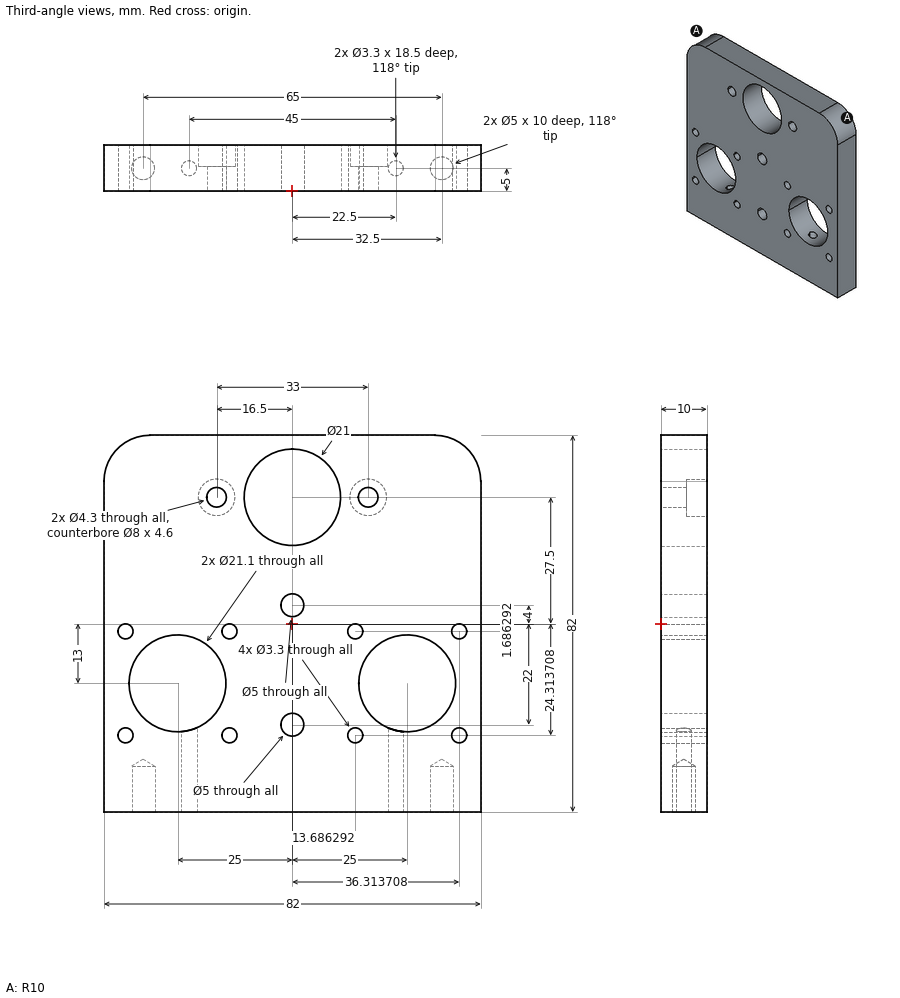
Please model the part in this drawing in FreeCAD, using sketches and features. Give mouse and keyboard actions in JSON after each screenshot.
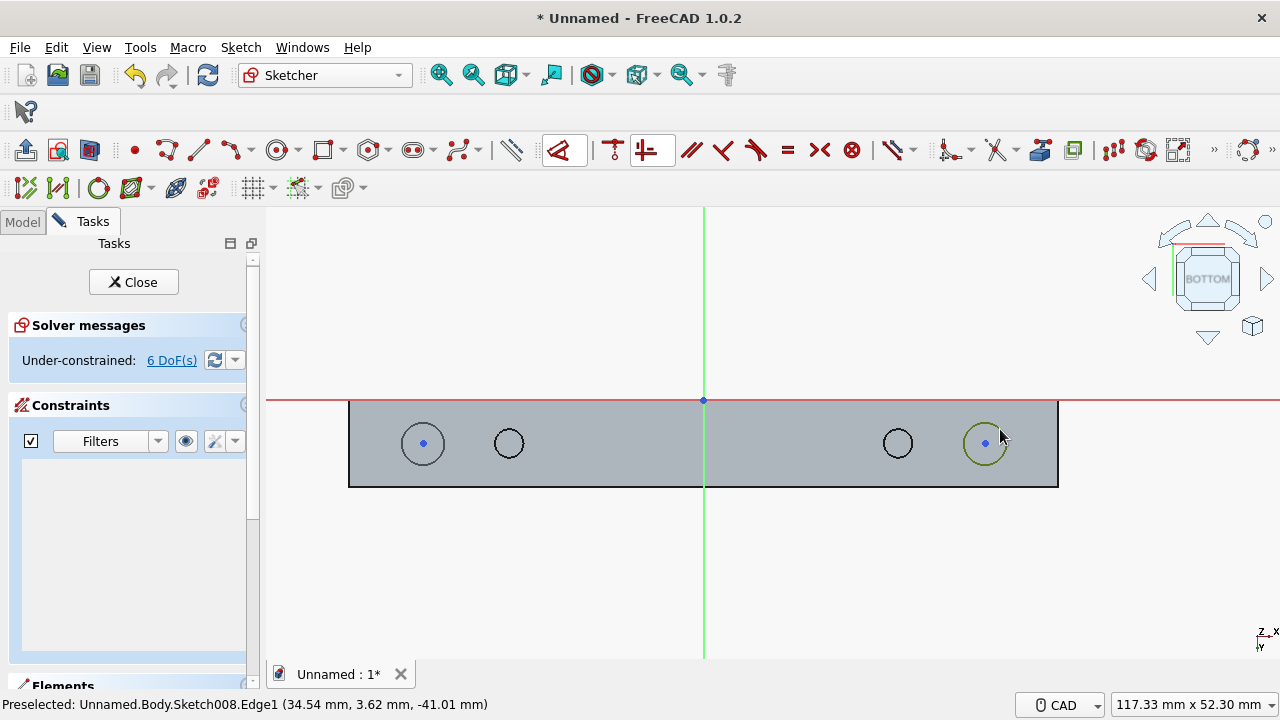
{"action": "left_click", "coordinate": [438, 429]}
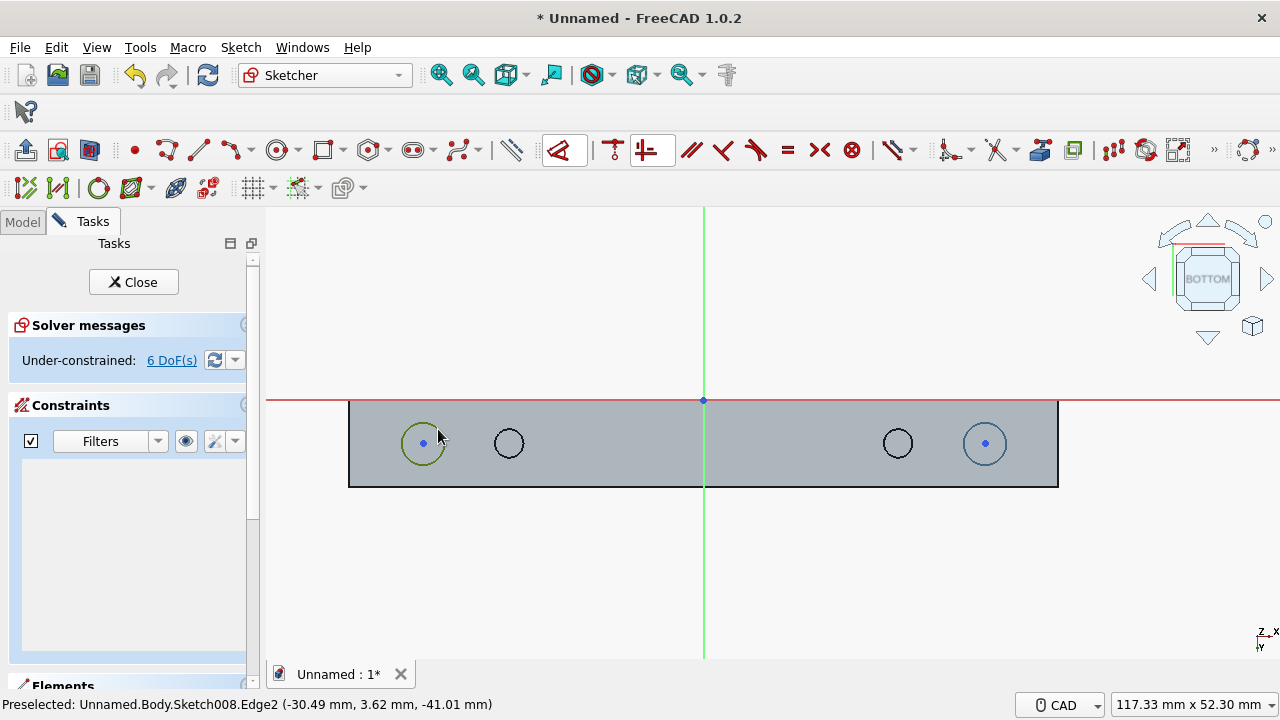
{"action": "left_click", "coordinate": [788, 150]}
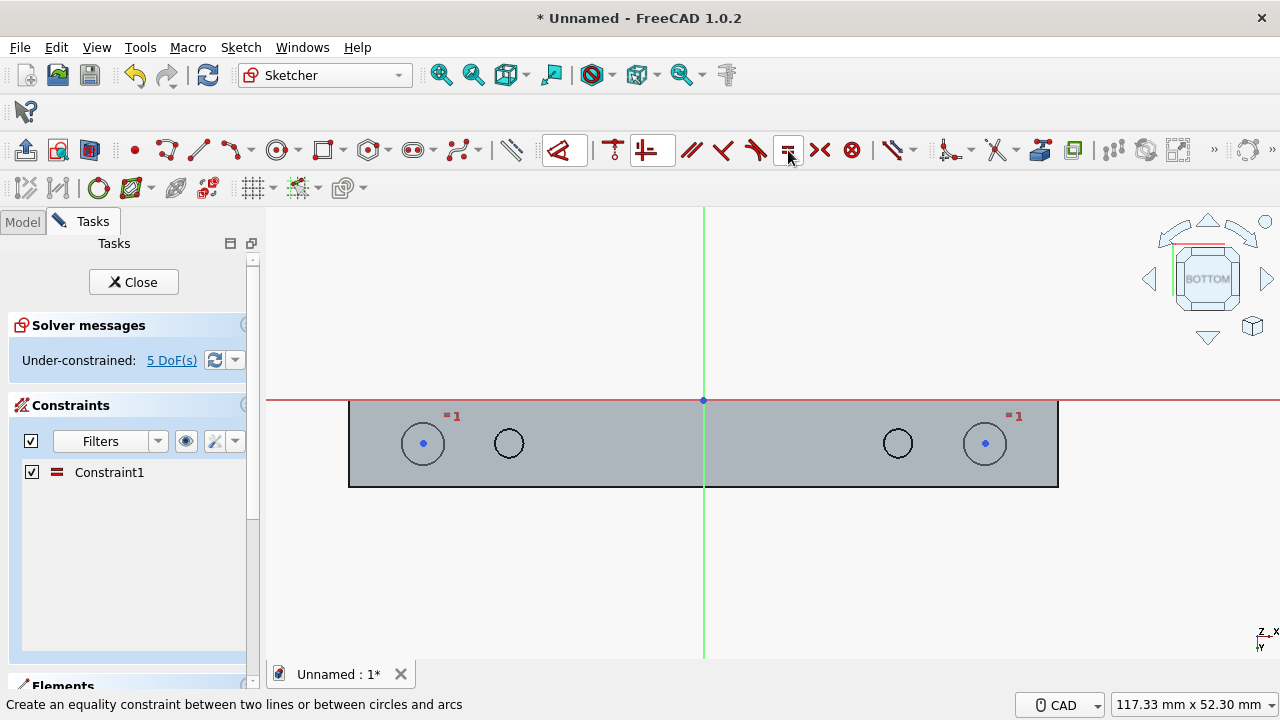
{"action": "left_click", "coordinate": [1000, 429]}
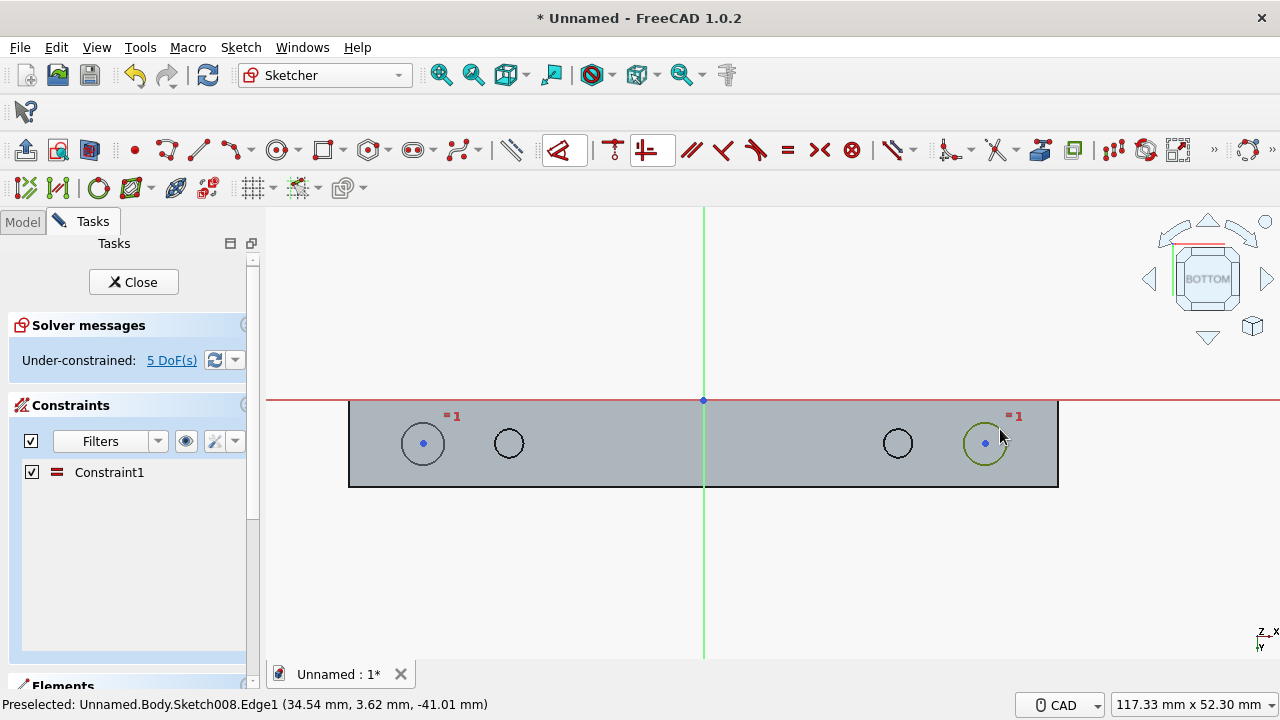
{"action": "left_click", "coordinate": [582, 150]}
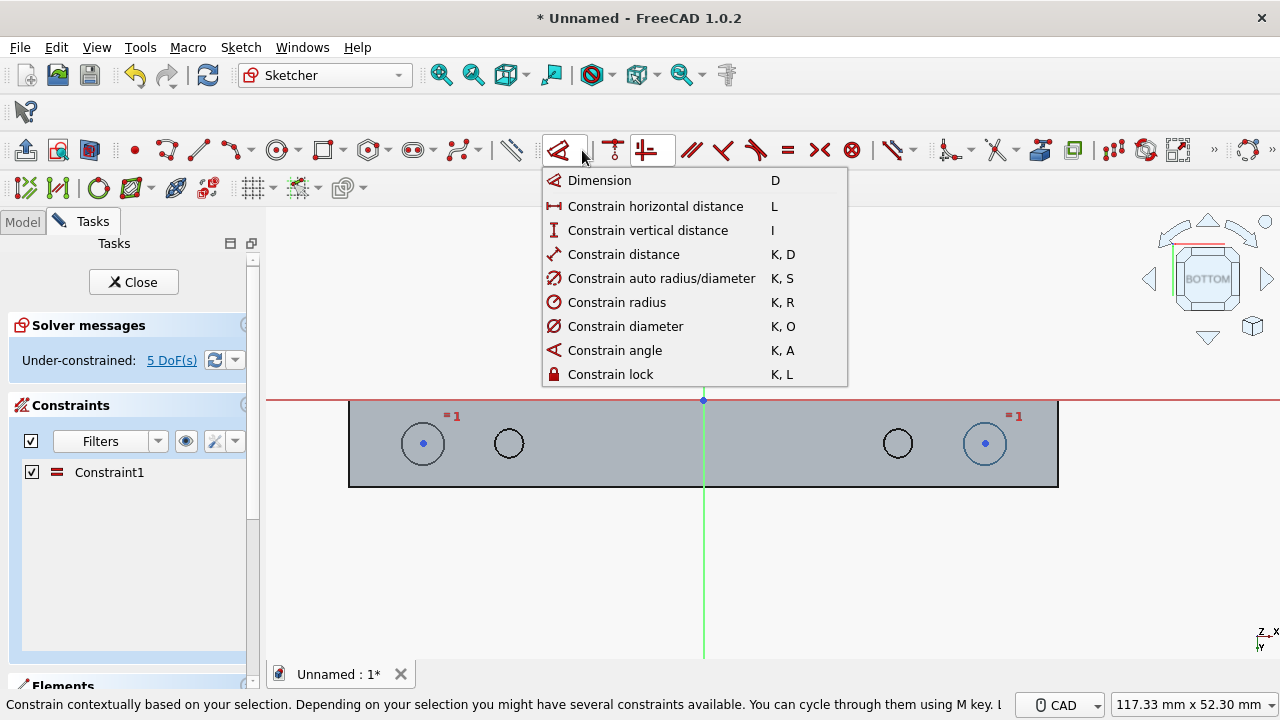
{"action": "left_click", "coordinate": [695, 326]}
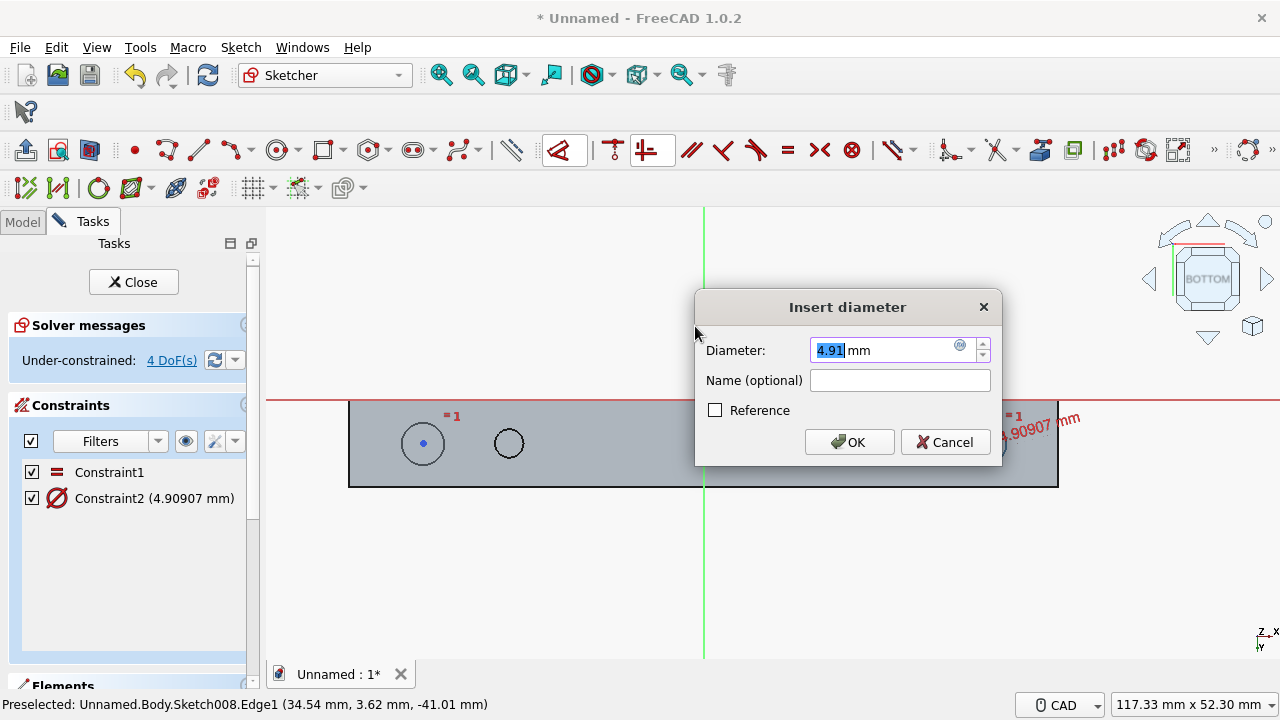
{"action": "type", "text": "5"}
{"action": "key", "text": "Return"}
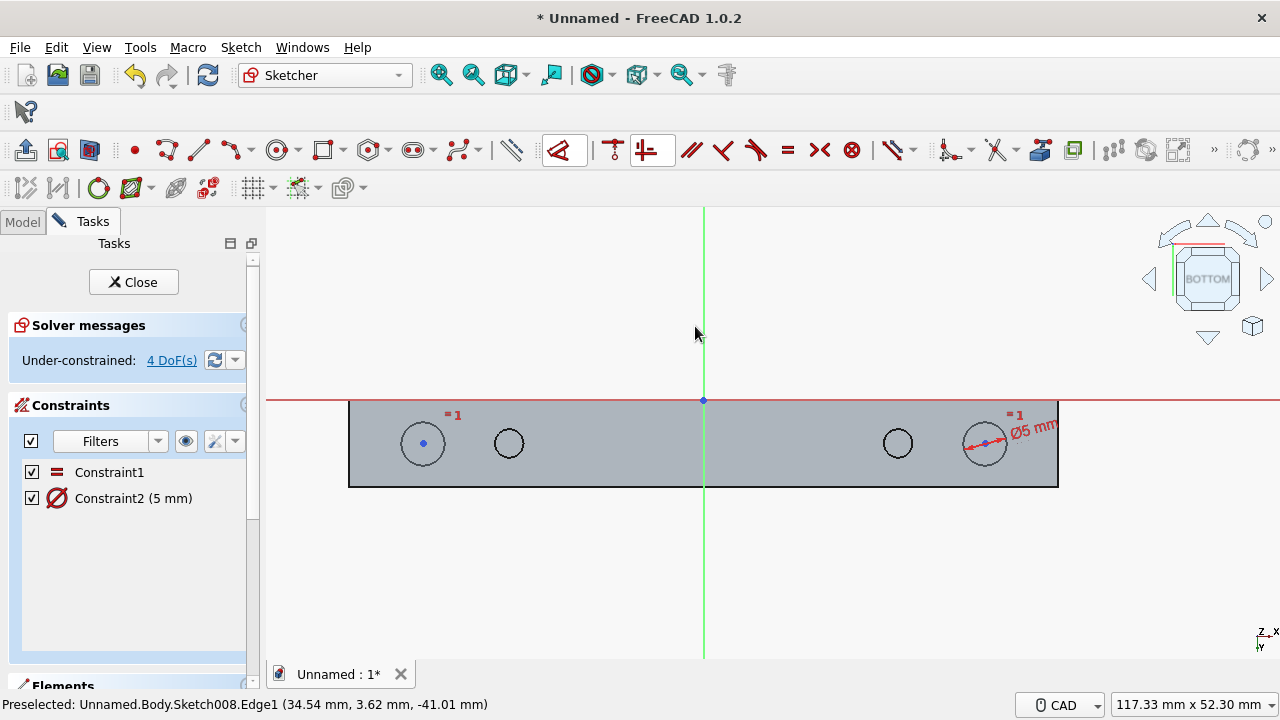
{"action": "left_click", "coordinate": [985, 444]}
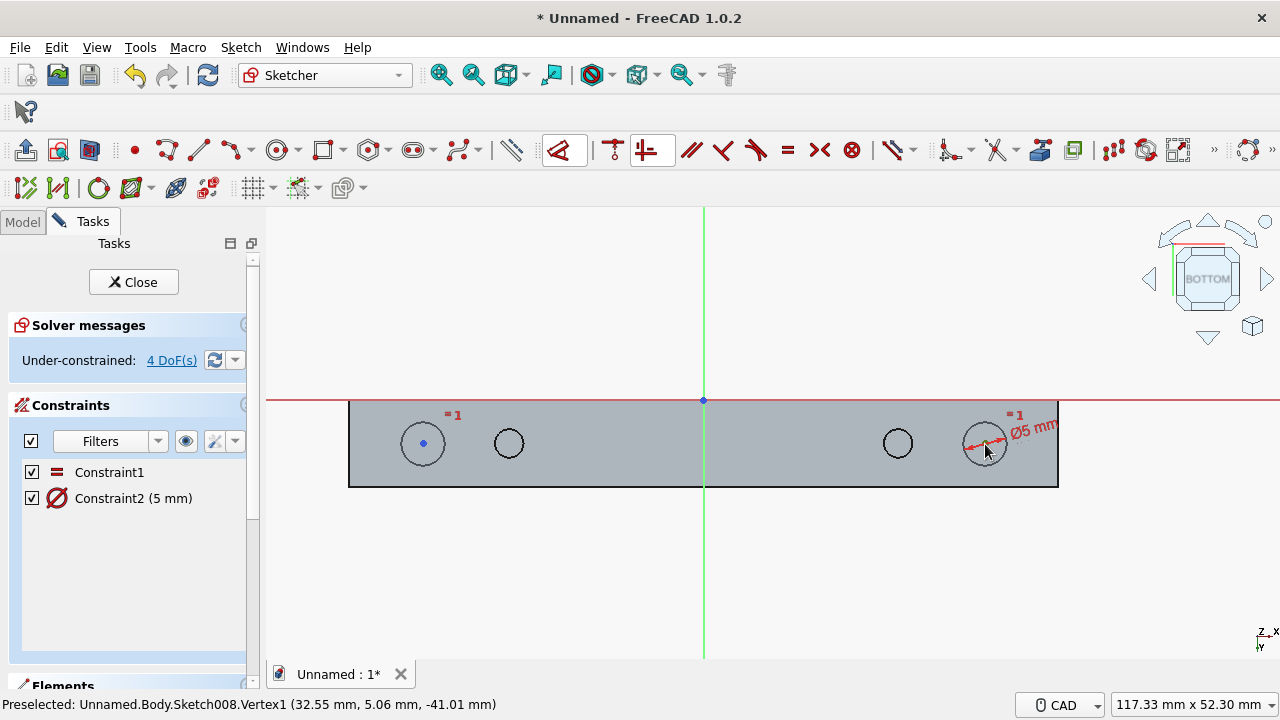
{"action": "key", "text": "i"}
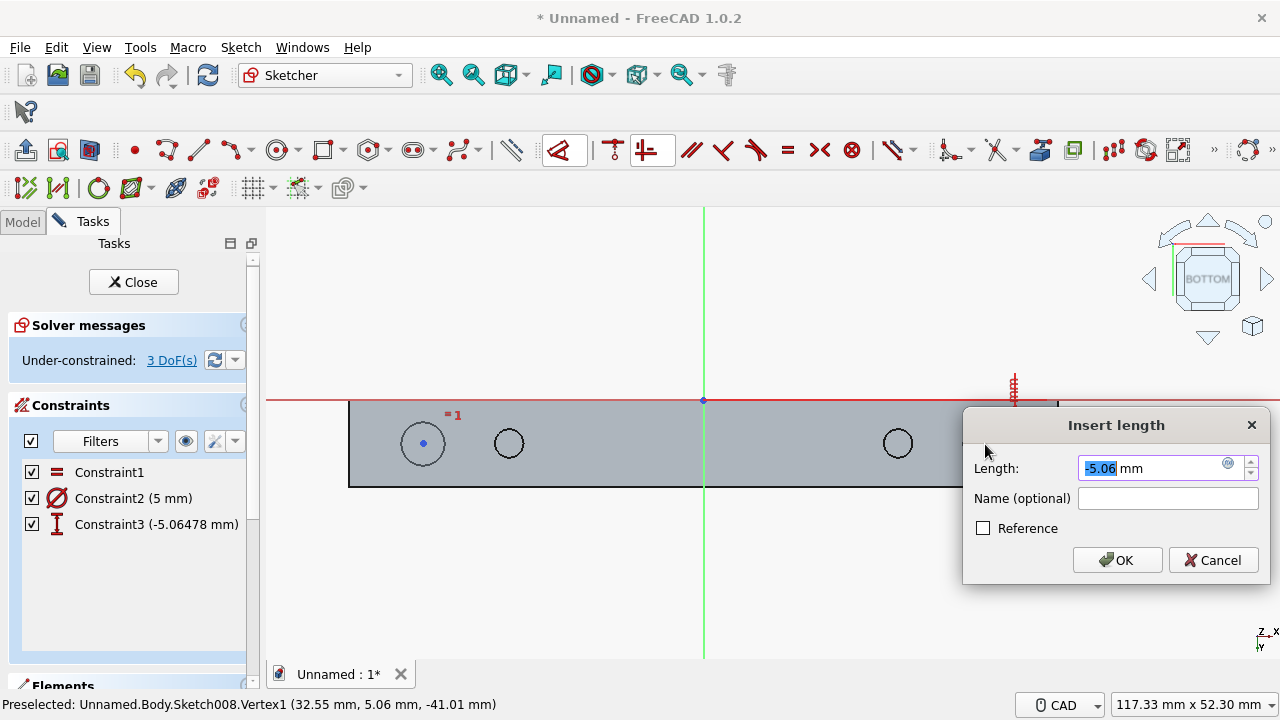
{"action": "type", "text": "-5"}
{"action": "key", "text": "Return"}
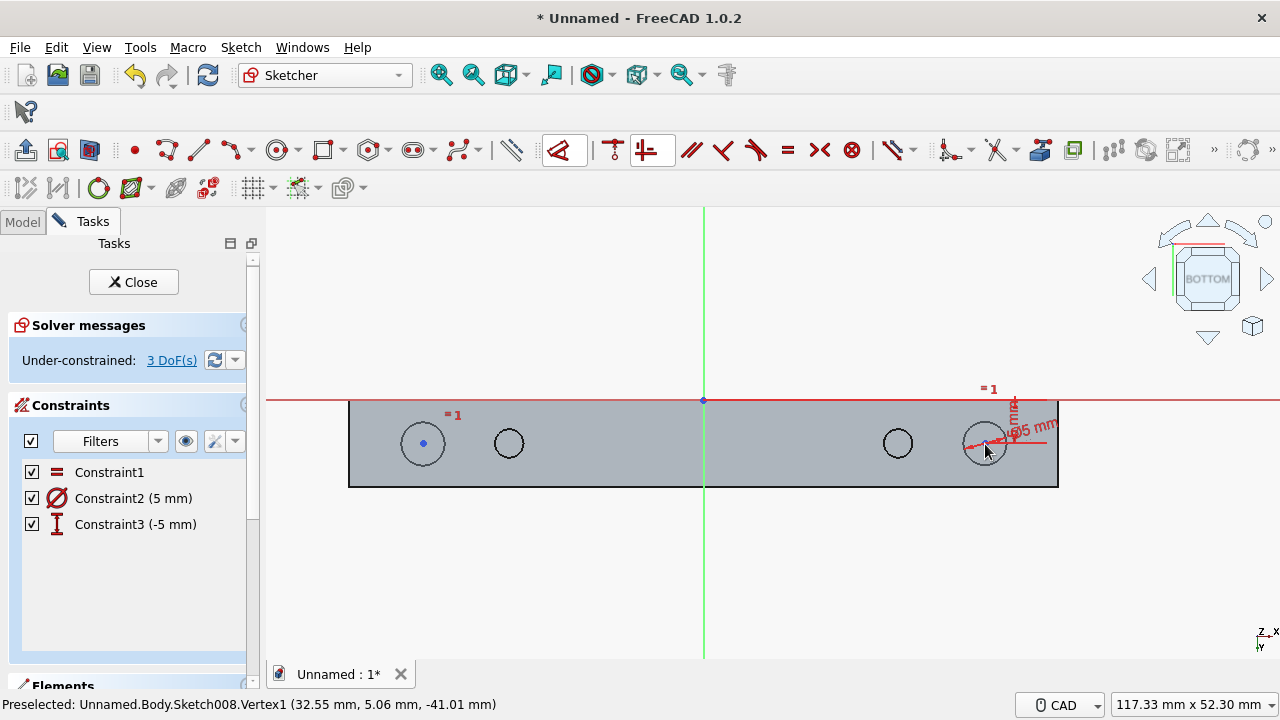
{"action": "left_click", "coordinate": [423, 444]}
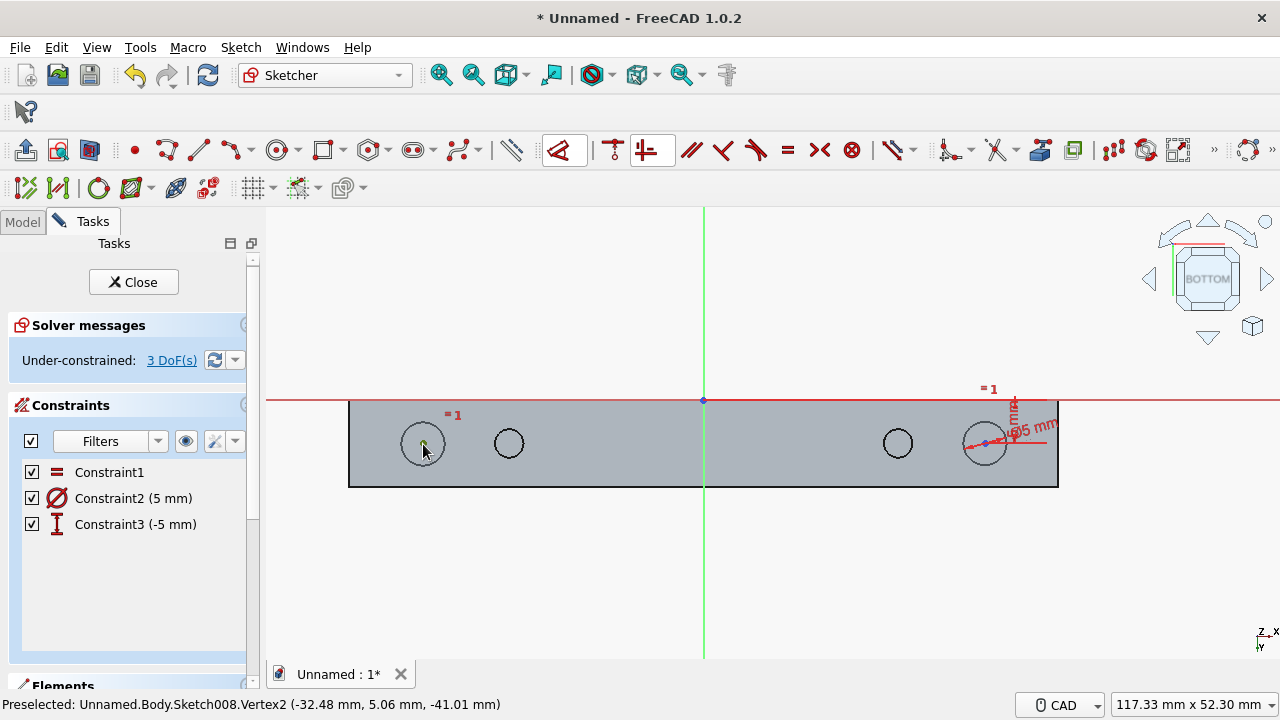
{"action": "left_click", "coordinate": [582, 150]}